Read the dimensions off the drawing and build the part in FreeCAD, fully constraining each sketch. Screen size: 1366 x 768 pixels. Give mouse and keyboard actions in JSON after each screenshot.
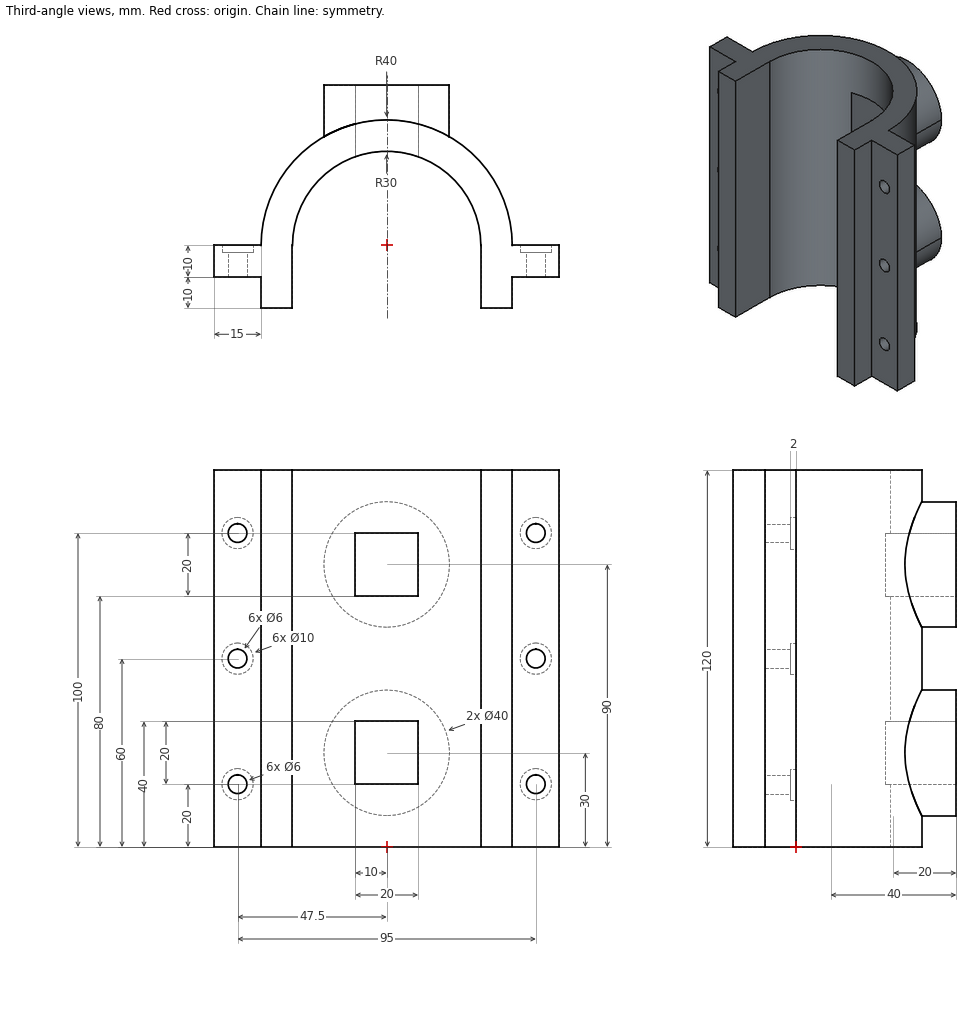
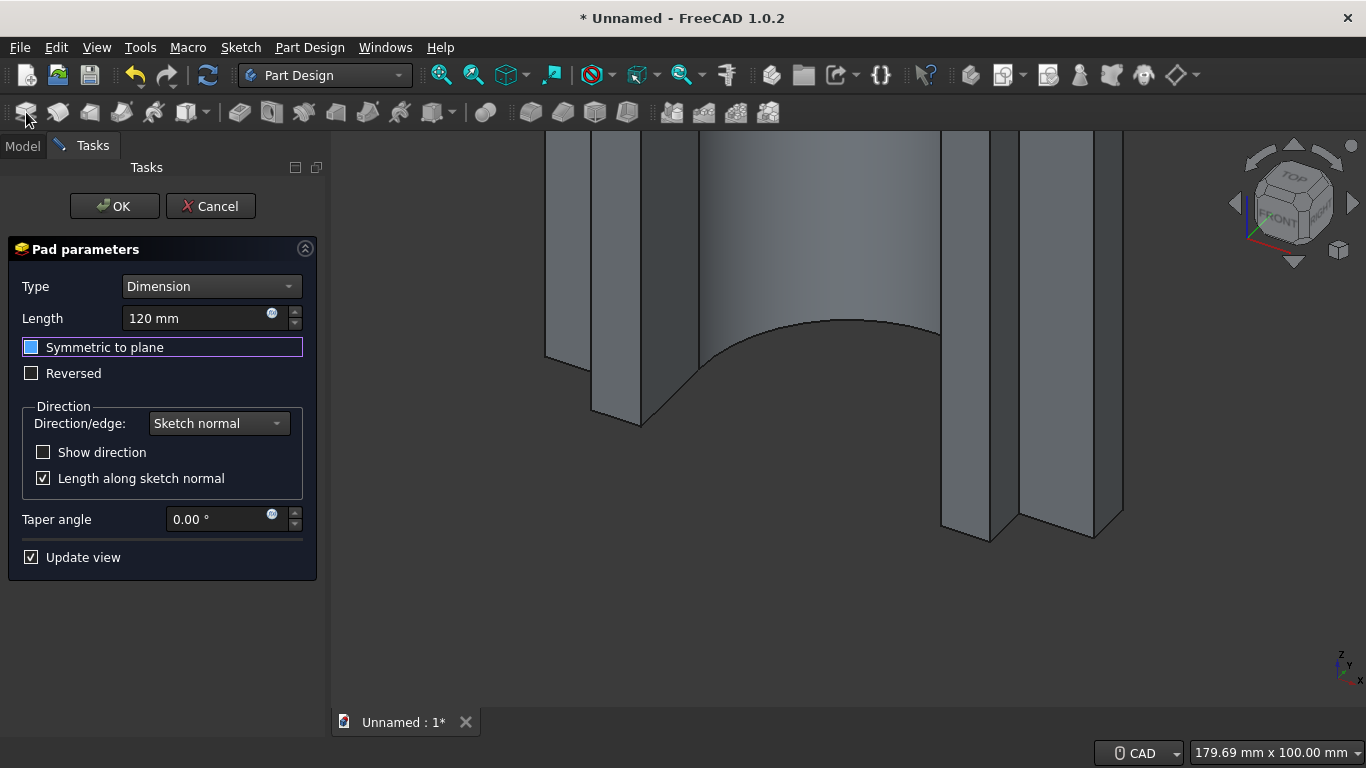
{"action": "left_click", "coordinate": [115, 206]}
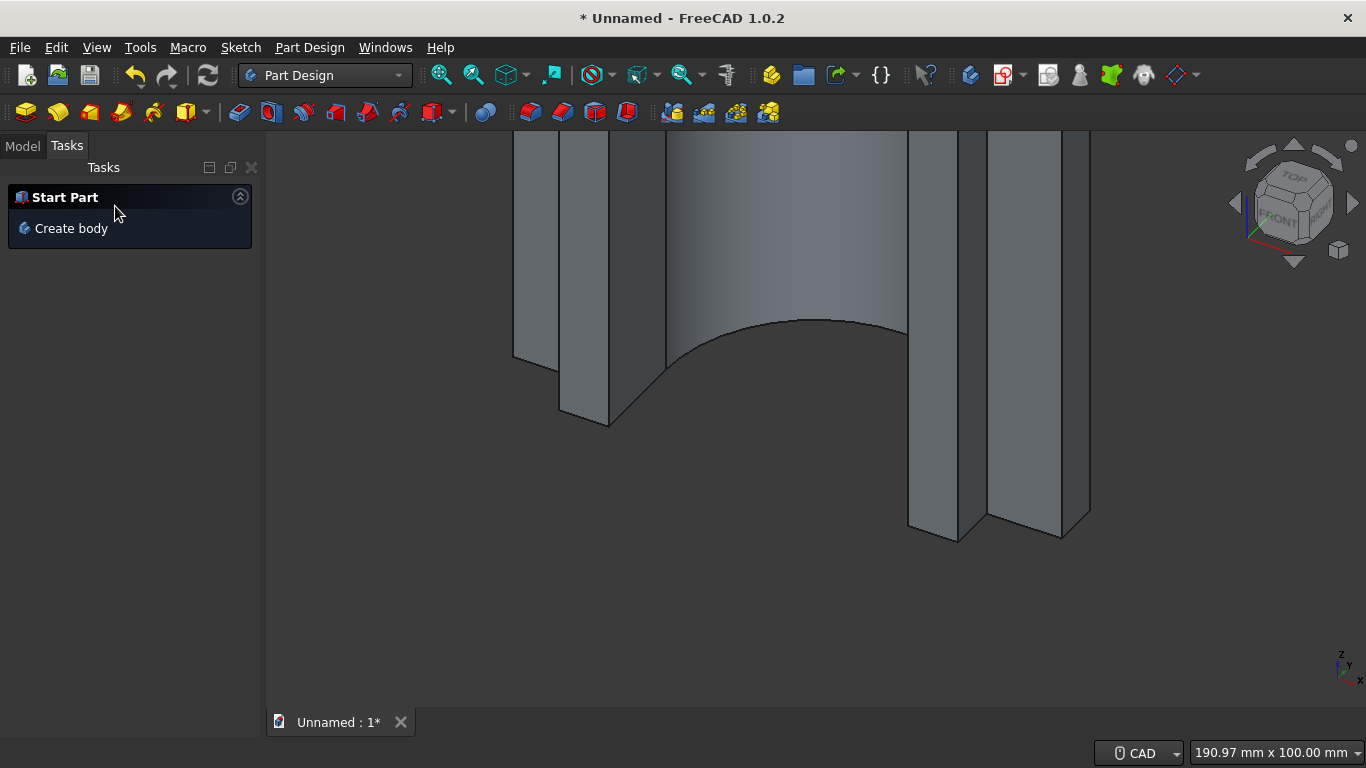
{"action": "left_click", "coordinate": [442, 76]}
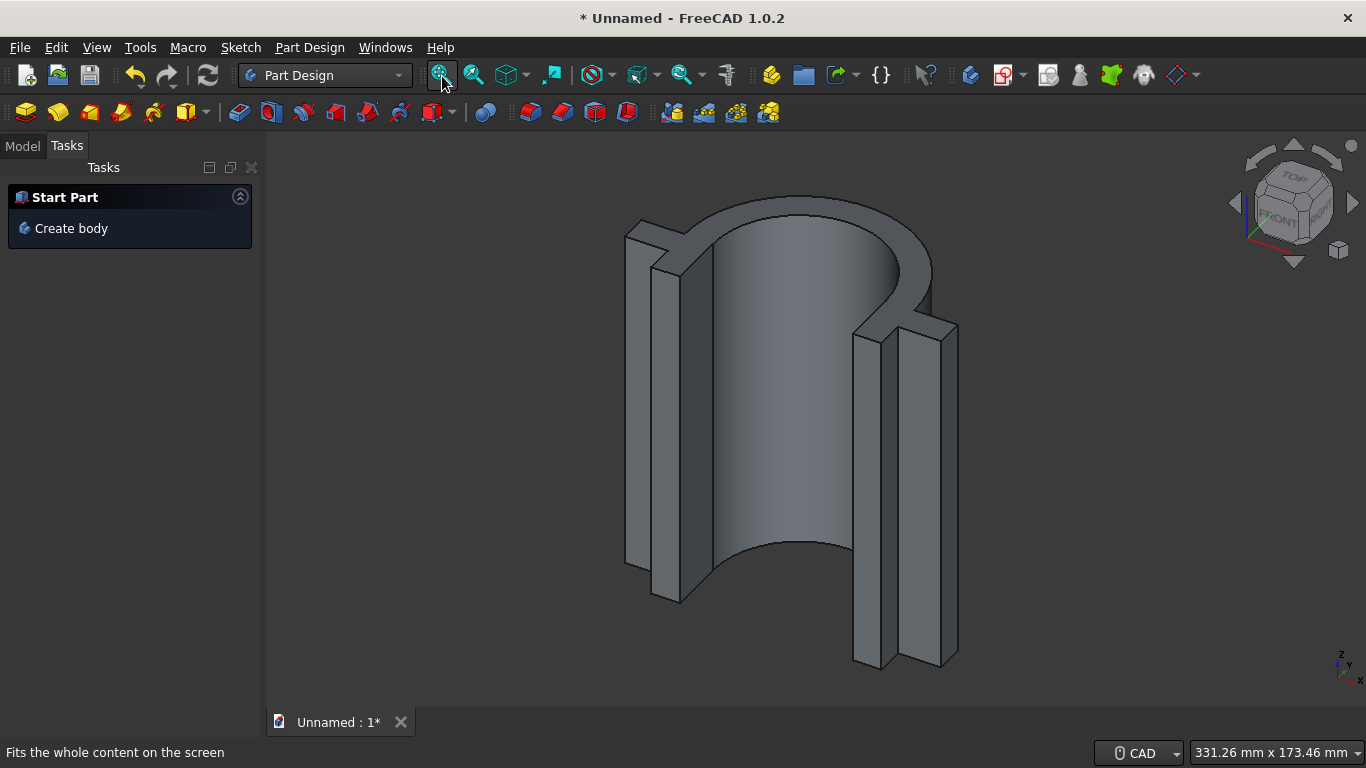
{"action": "left_click", "coordinate": [1004, 76]}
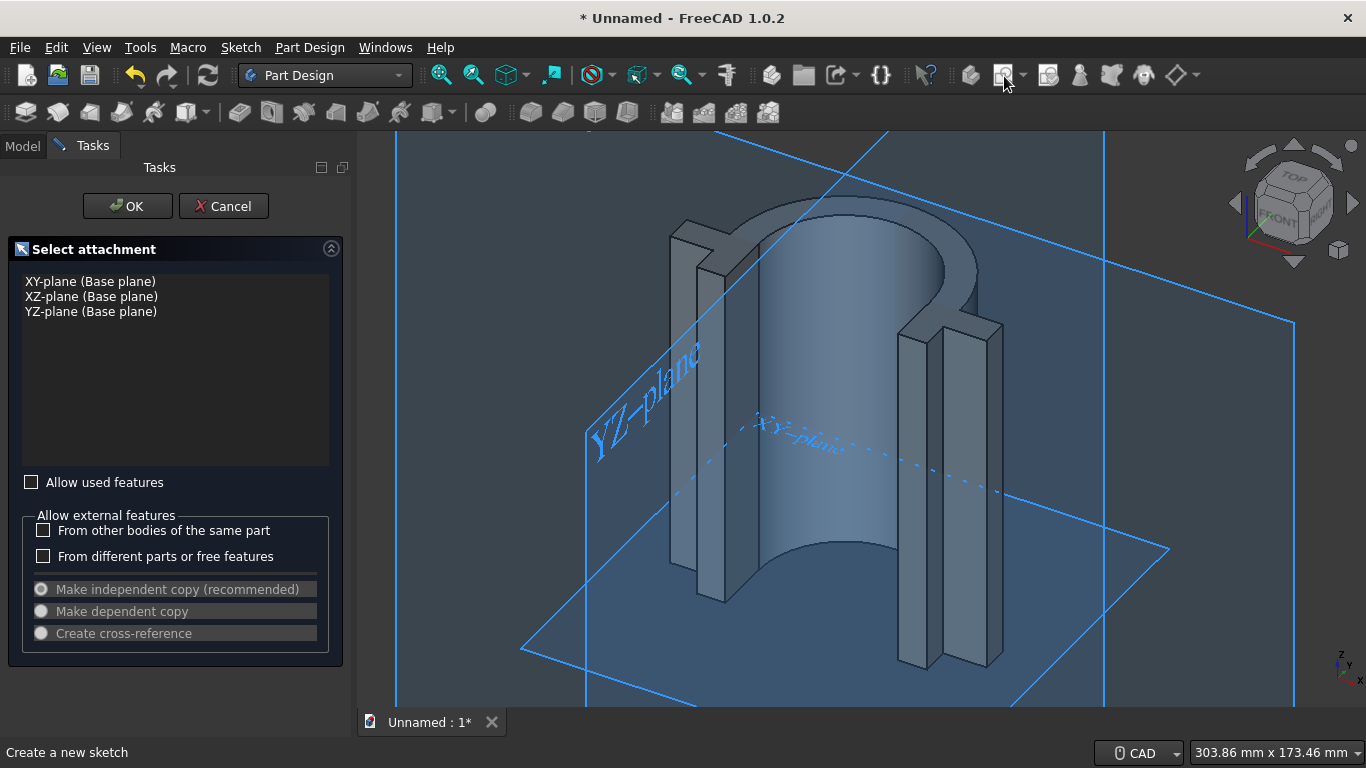
{"action": "left_click", "coordinate": [82, 296]}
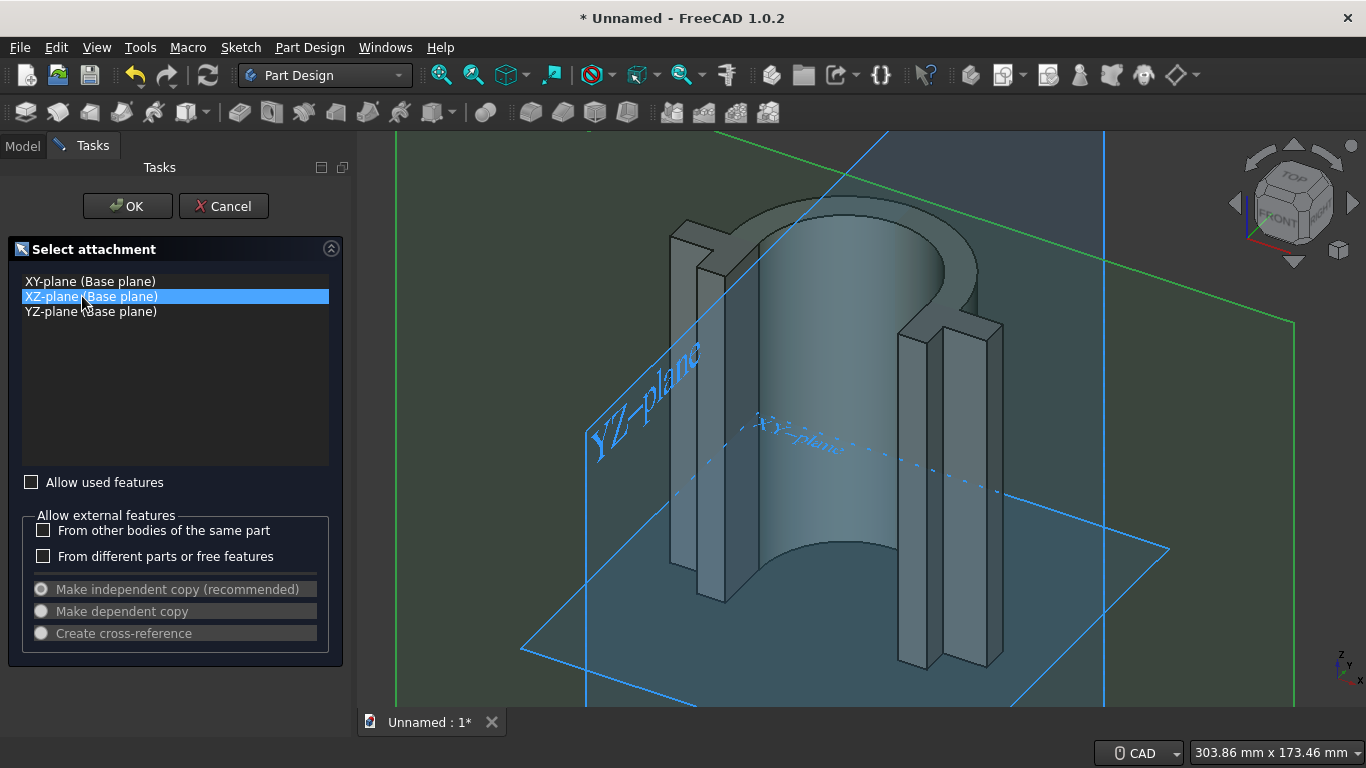
{"action": "left_click", "coordinate": [128, 206]}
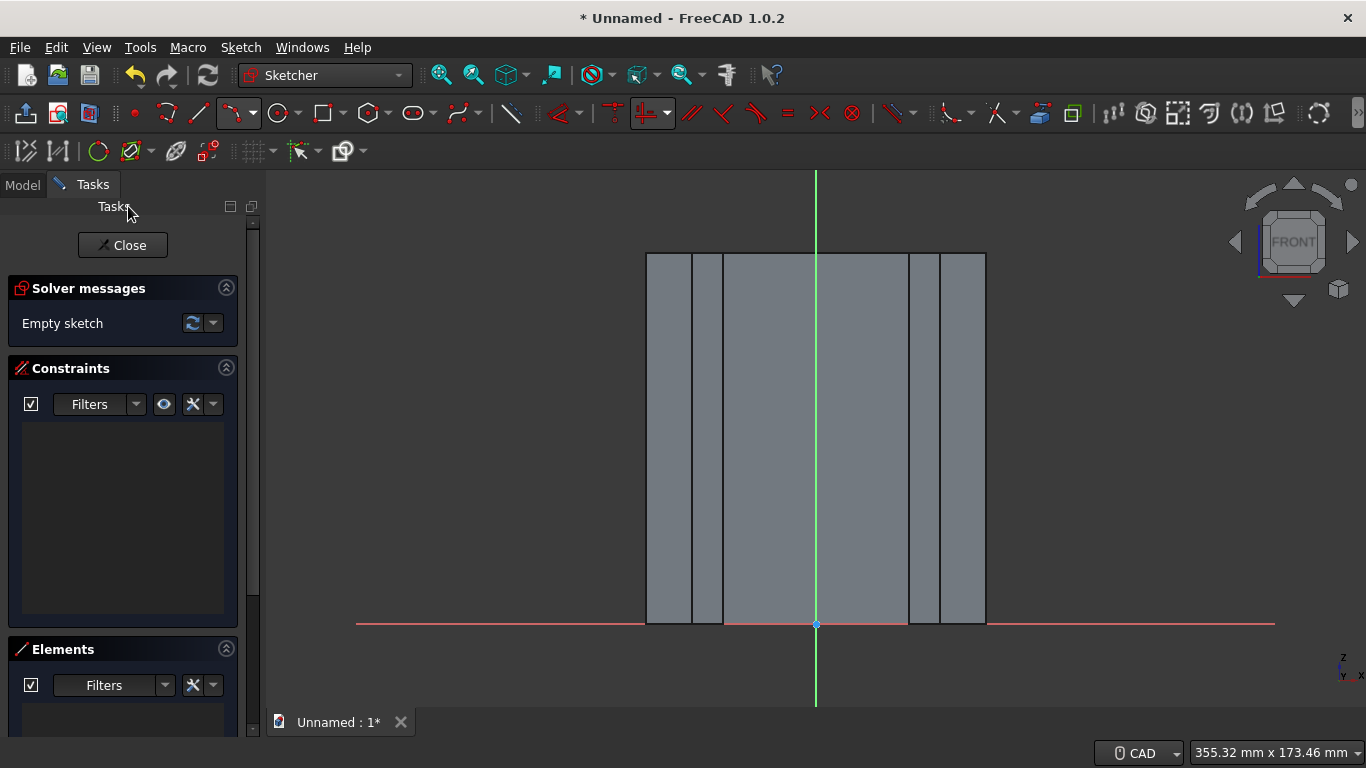
{"action": "left_click", "coordinate": [90, 114]}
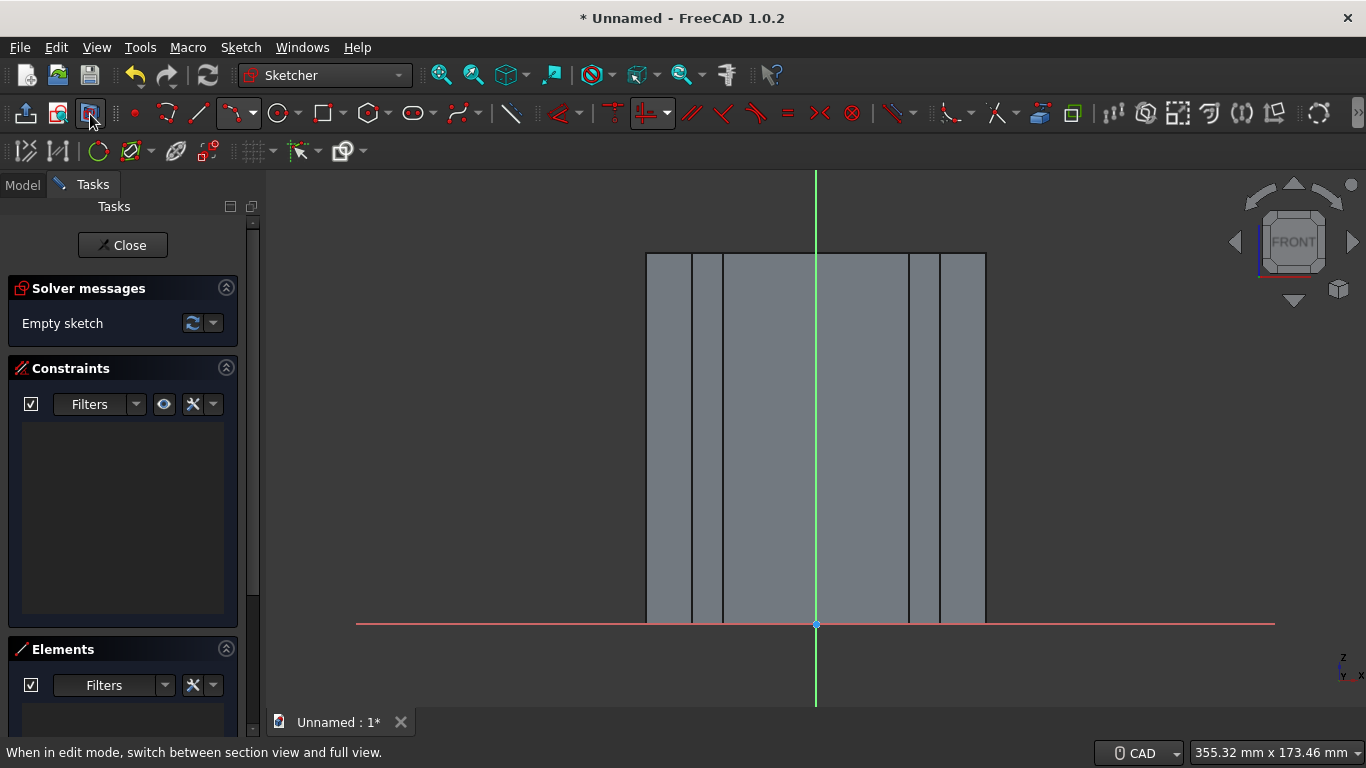
{"action": "left_click", "coordinate": [278, 114]}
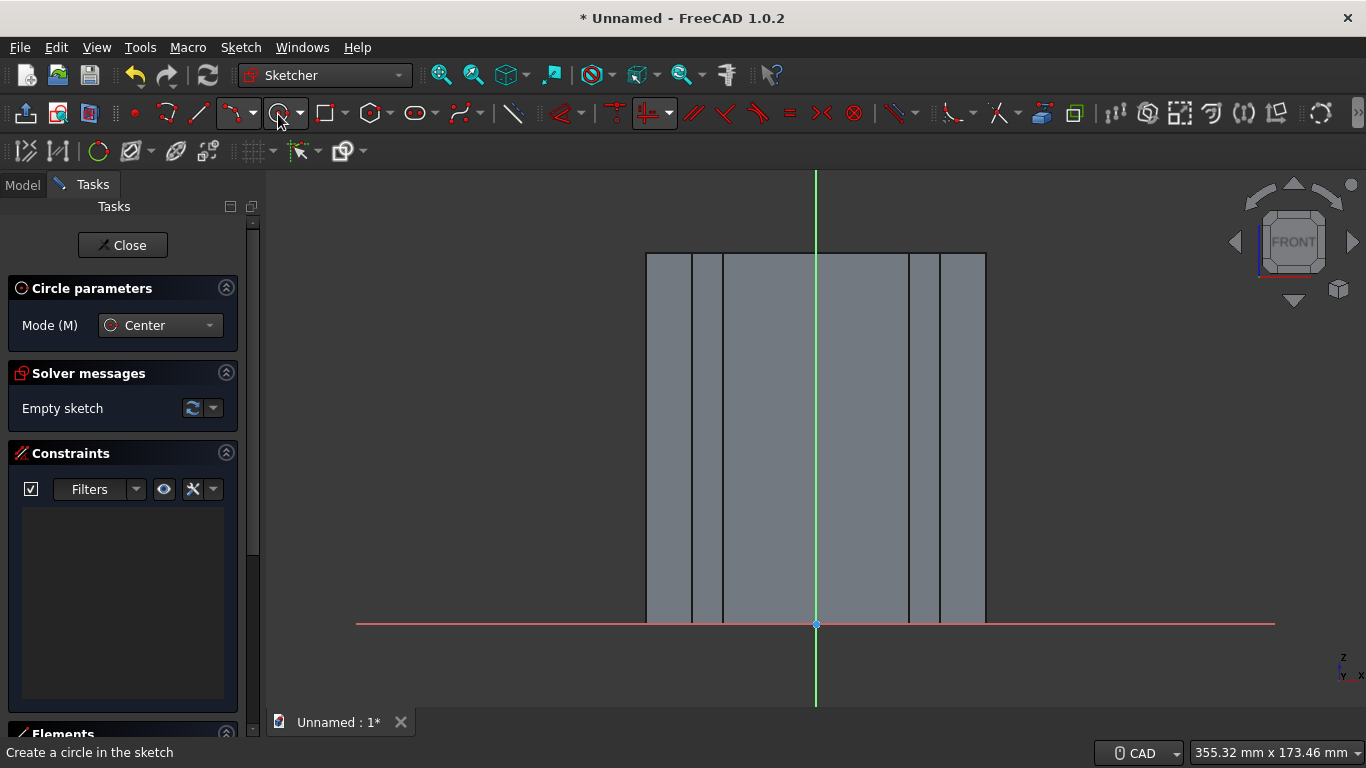
{"action": "scroll", "coordinate": [669, 562], "scroll_direction": "up", "scroll_amount": 5}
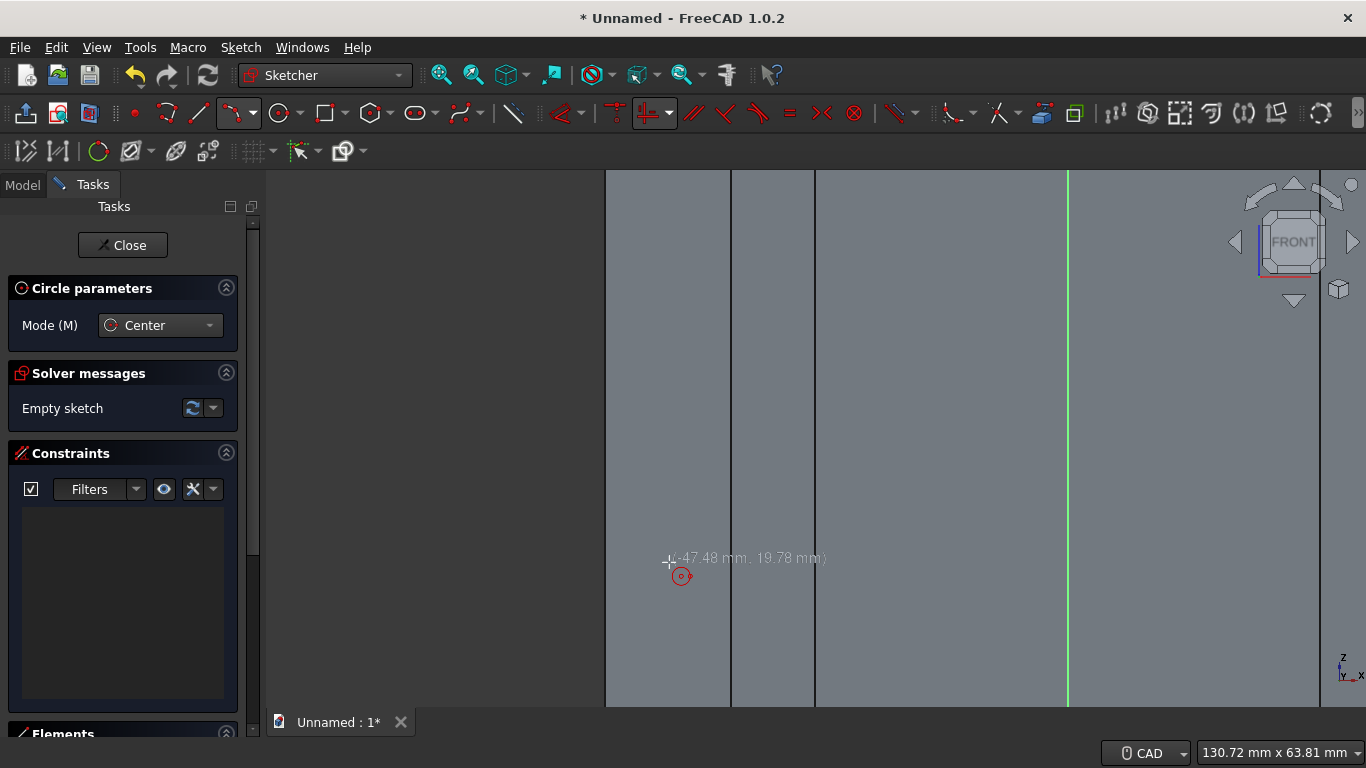
{"action": "left_click", "coordinate": [668, 562]}
{"action": "left_click", "coordinate": [686, 544]}